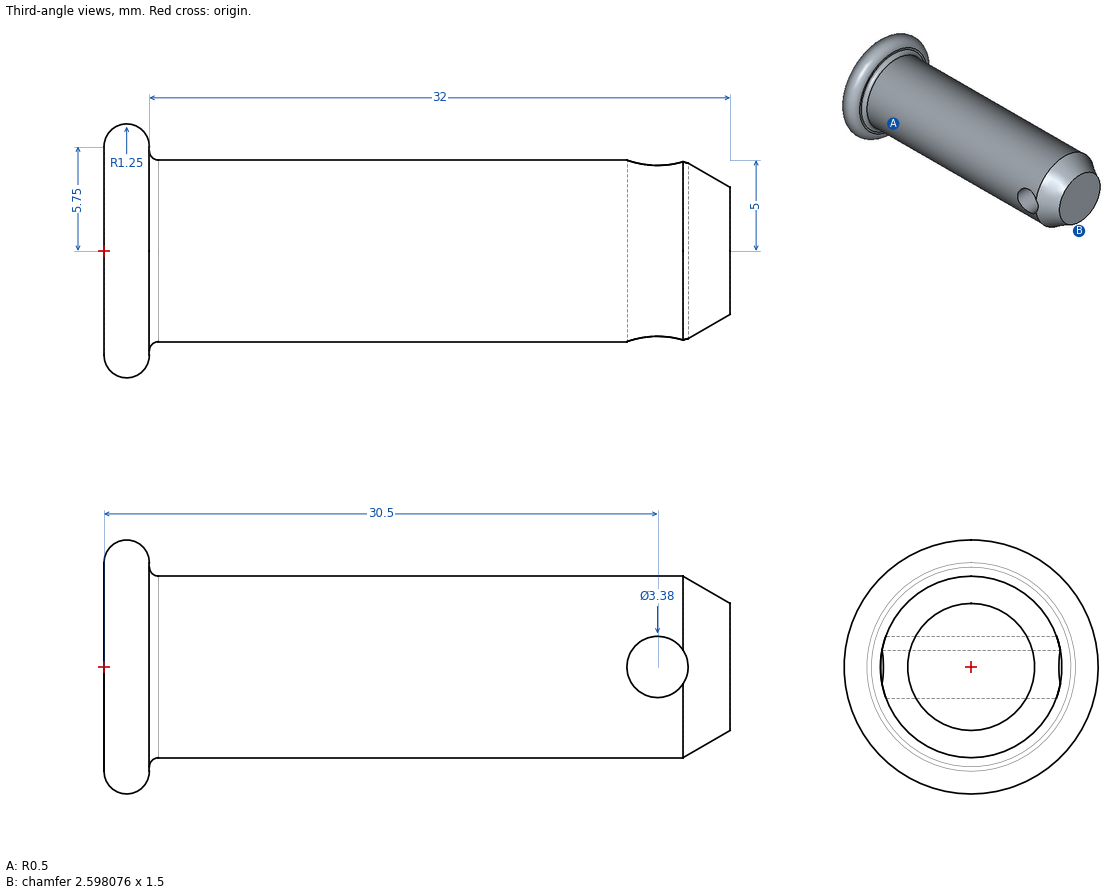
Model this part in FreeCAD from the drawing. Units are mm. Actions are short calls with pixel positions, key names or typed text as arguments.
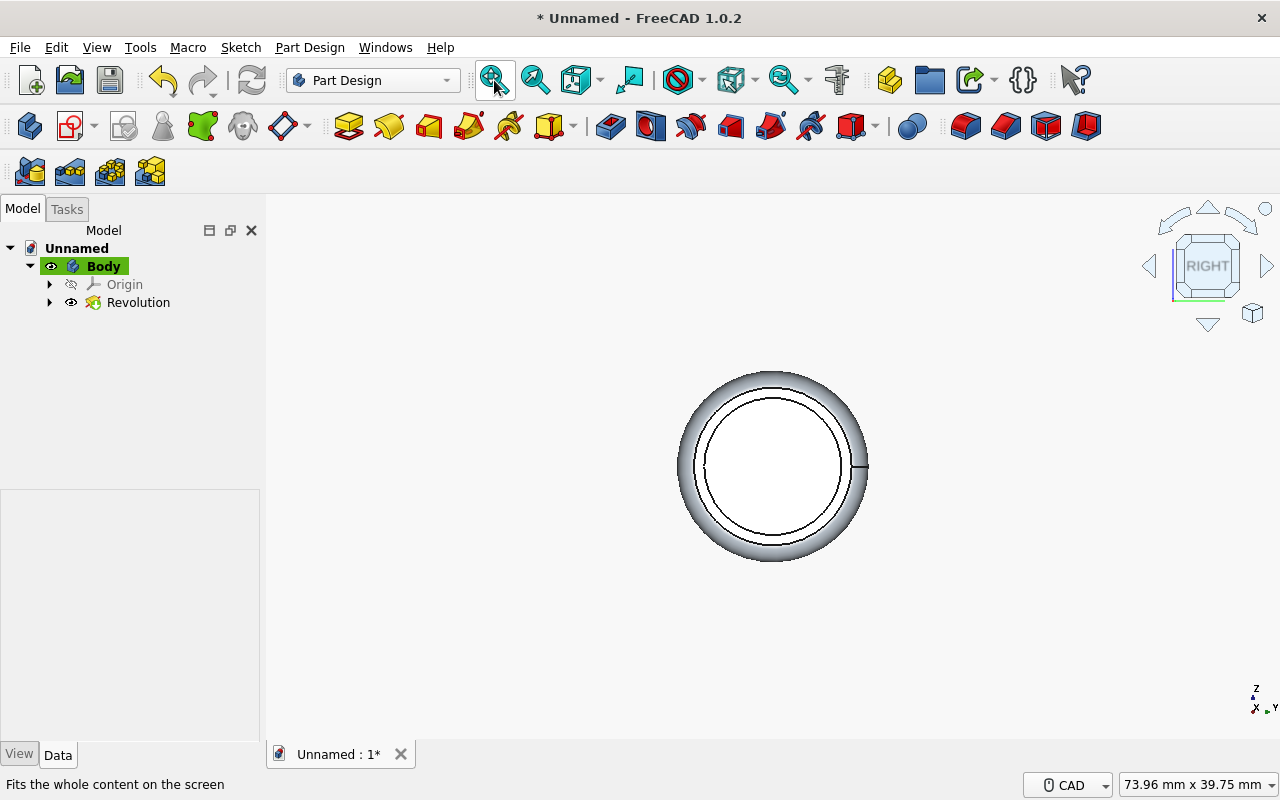
key(5)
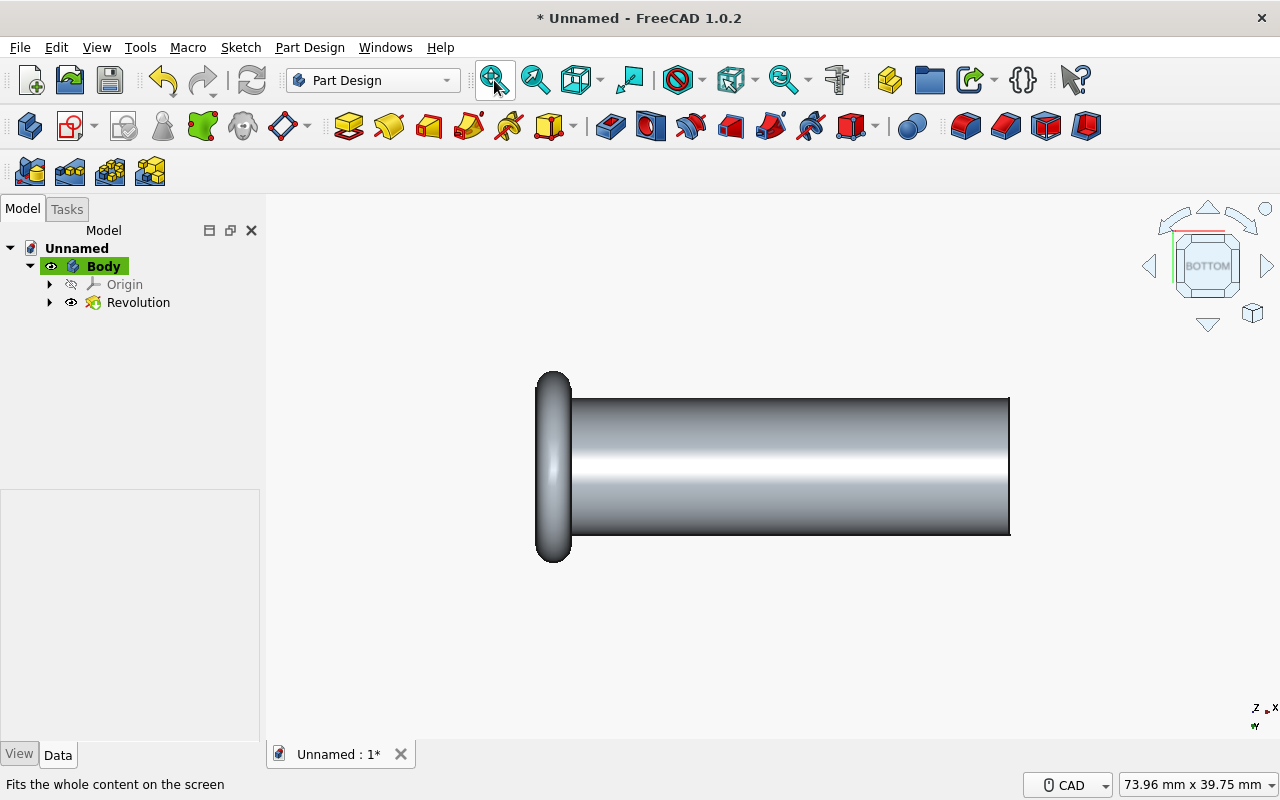
key(4)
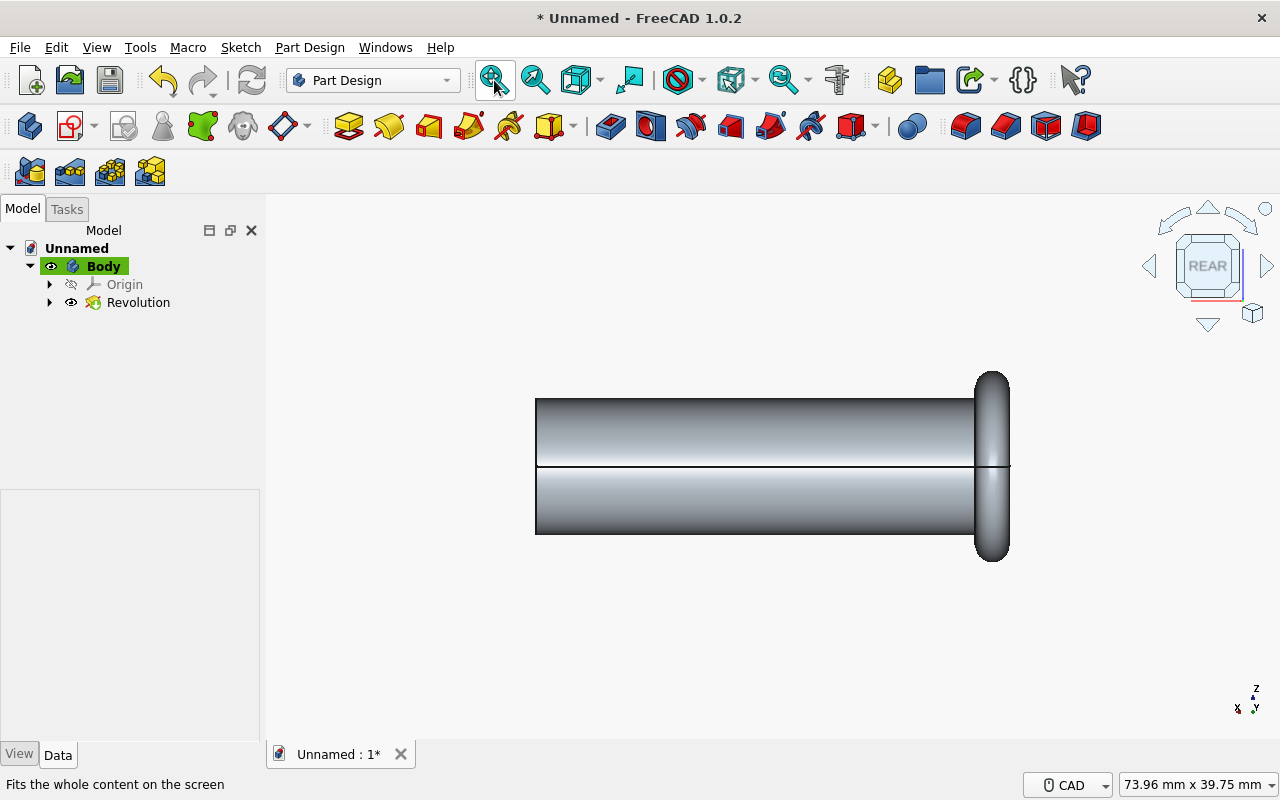
key(6)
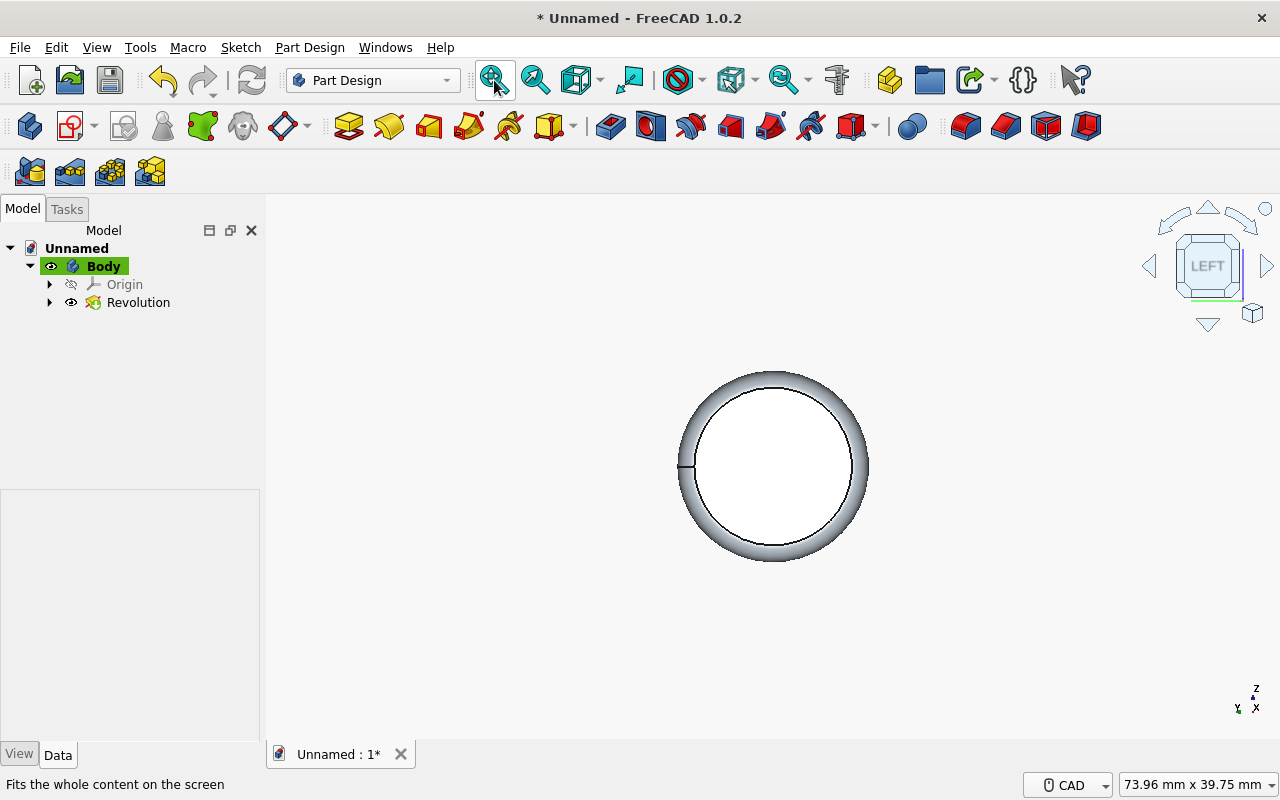
key(v)
key(f)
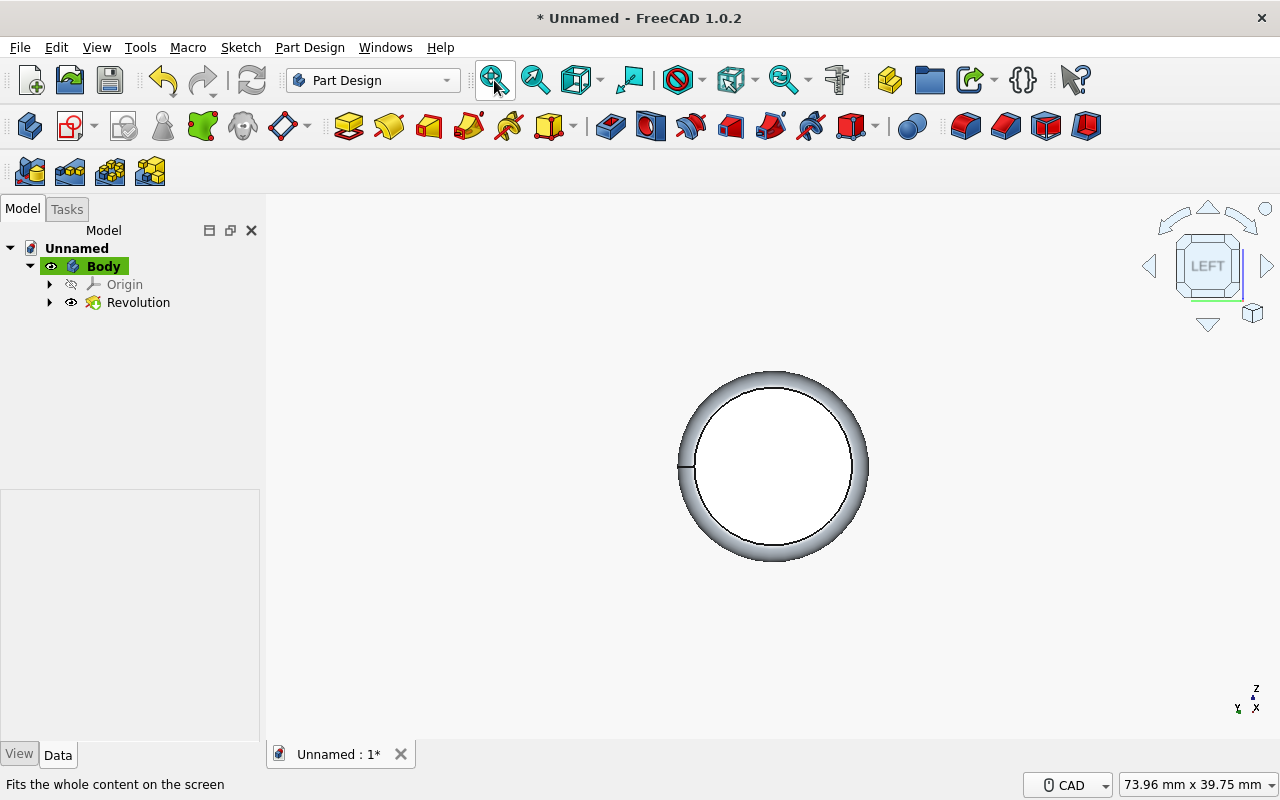
key(v)
key(3)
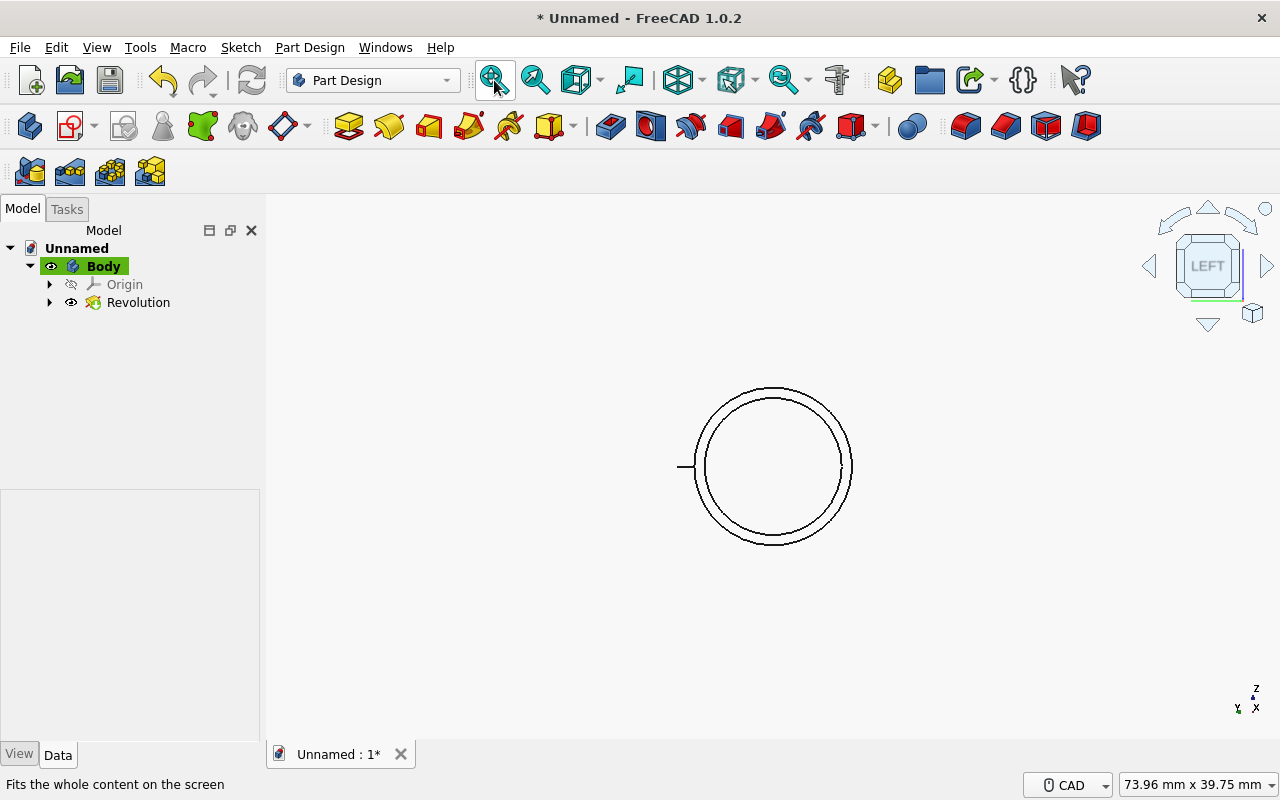
key(0)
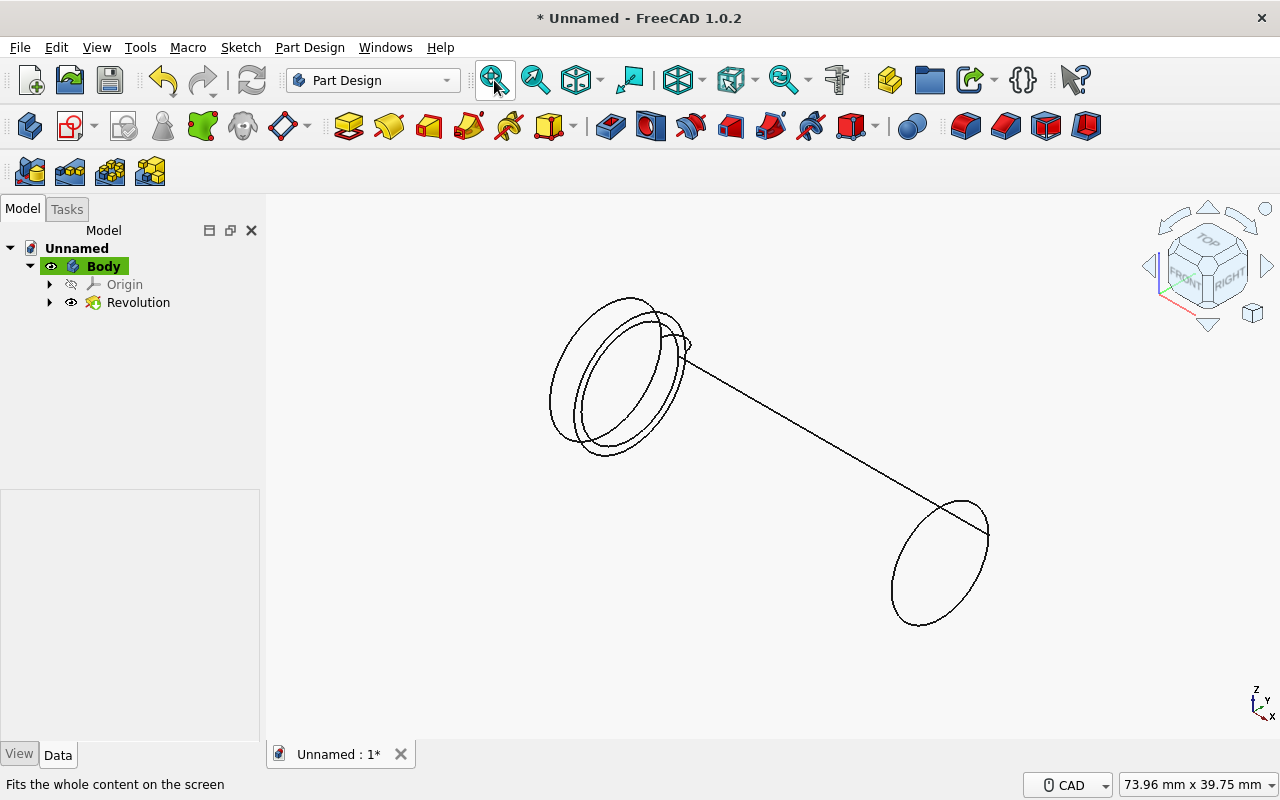
click(581, 411)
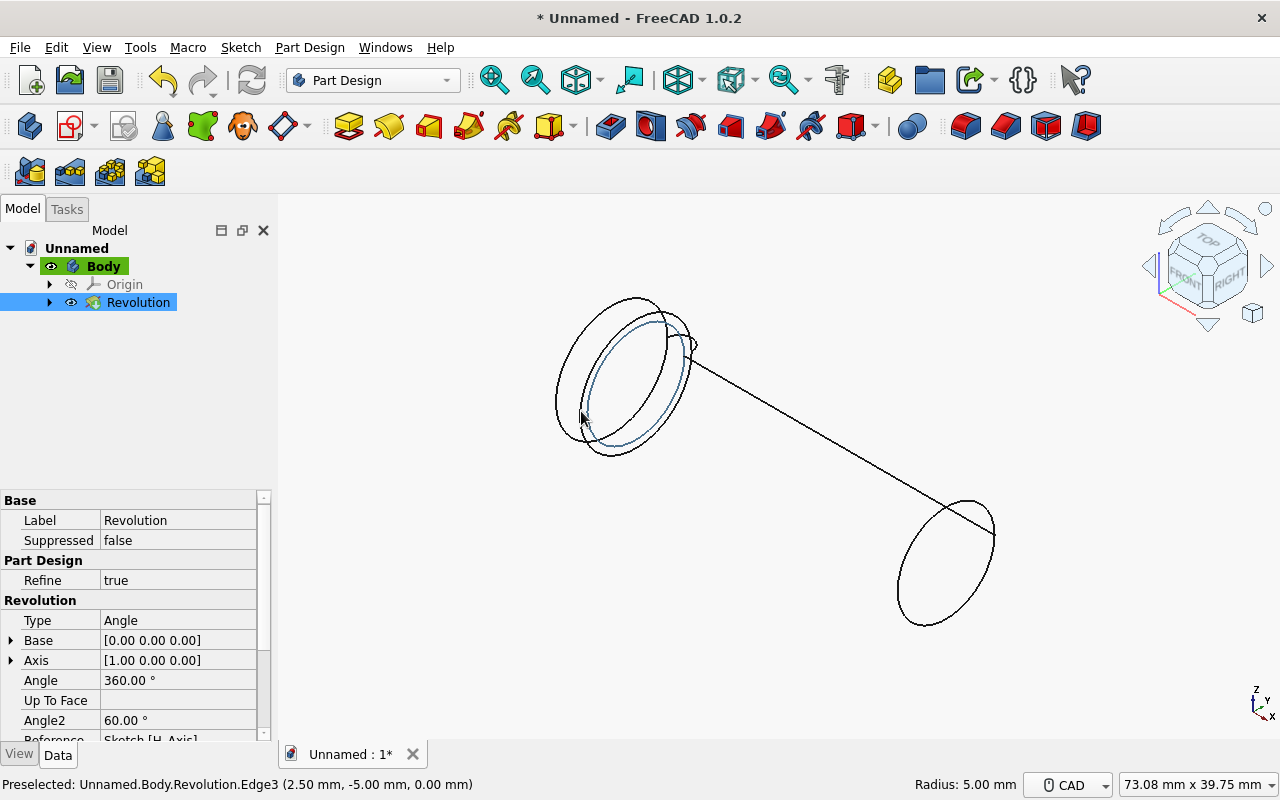
key(v)
key(1)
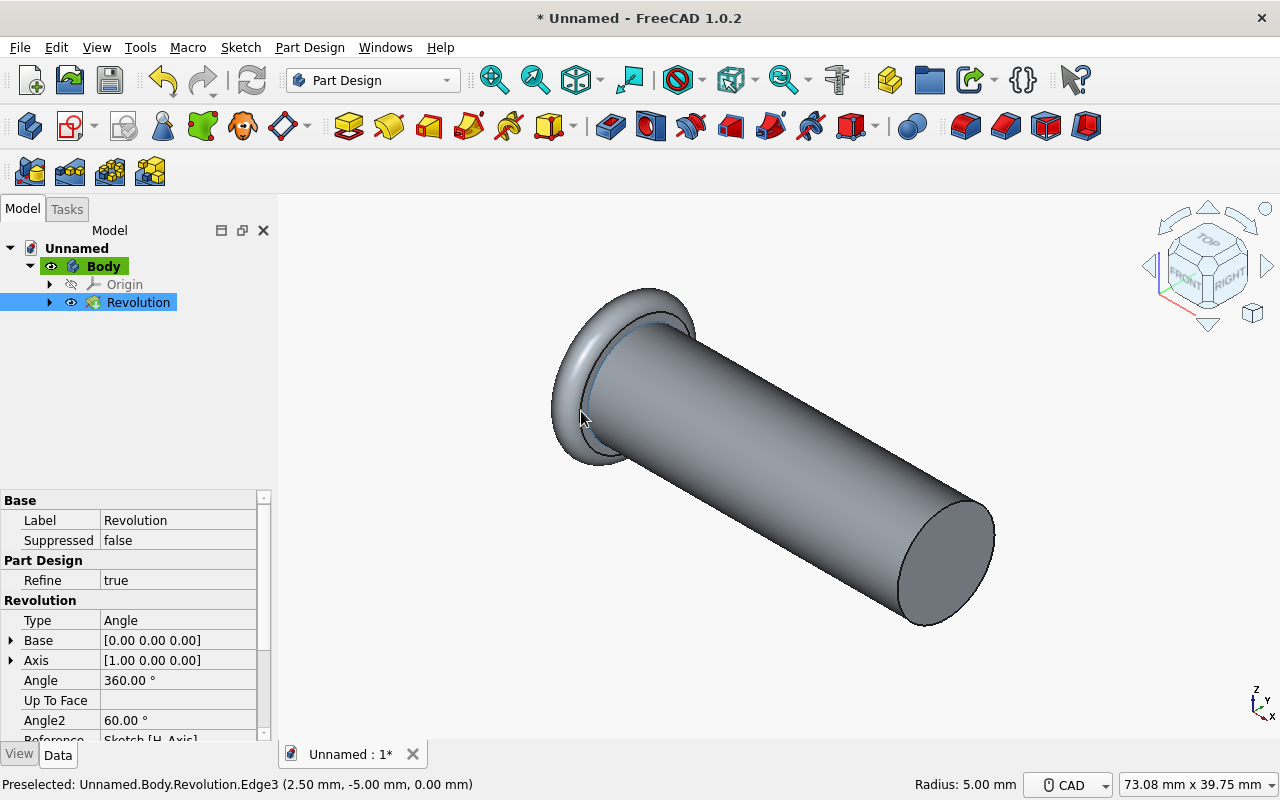
click(966, 126)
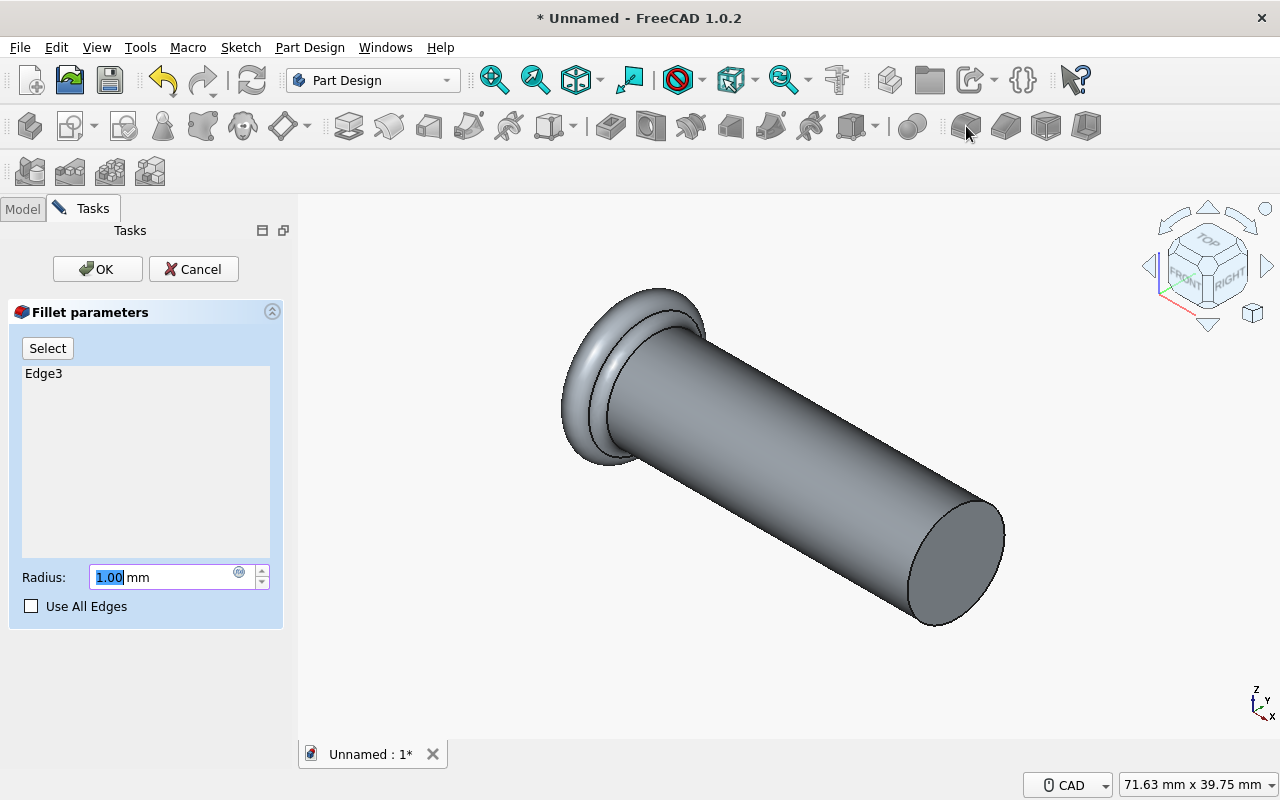
text(0.5)
key(Tab)